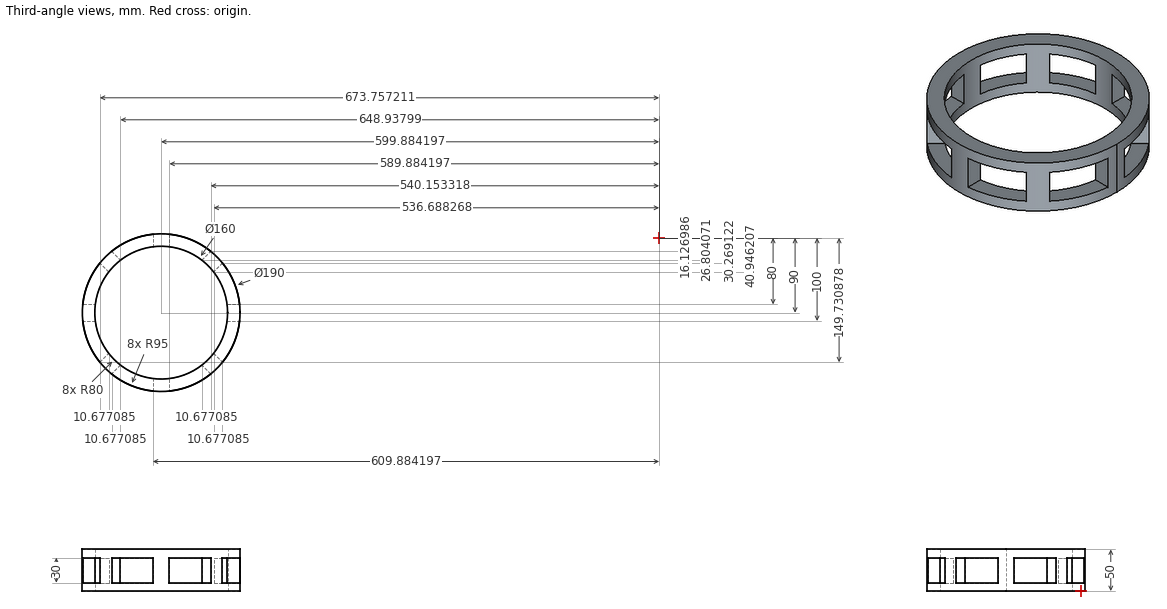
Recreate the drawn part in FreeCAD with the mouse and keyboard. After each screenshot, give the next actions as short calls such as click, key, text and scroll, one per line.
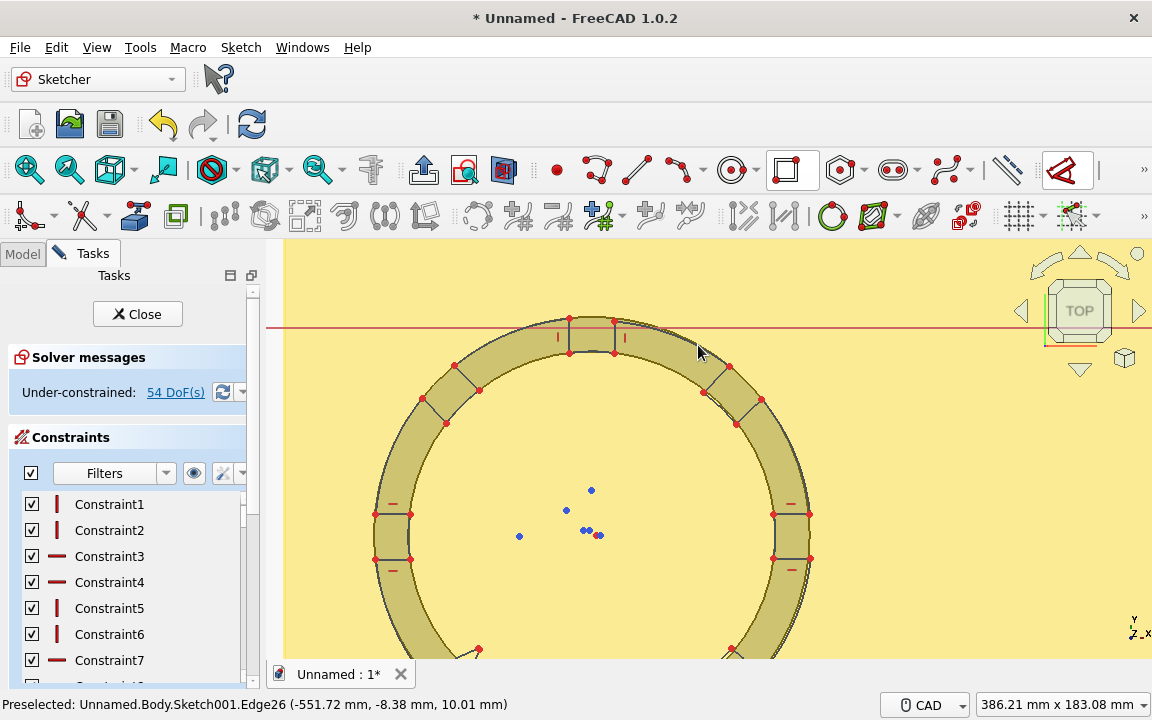
scroll(700, 345, down, 3)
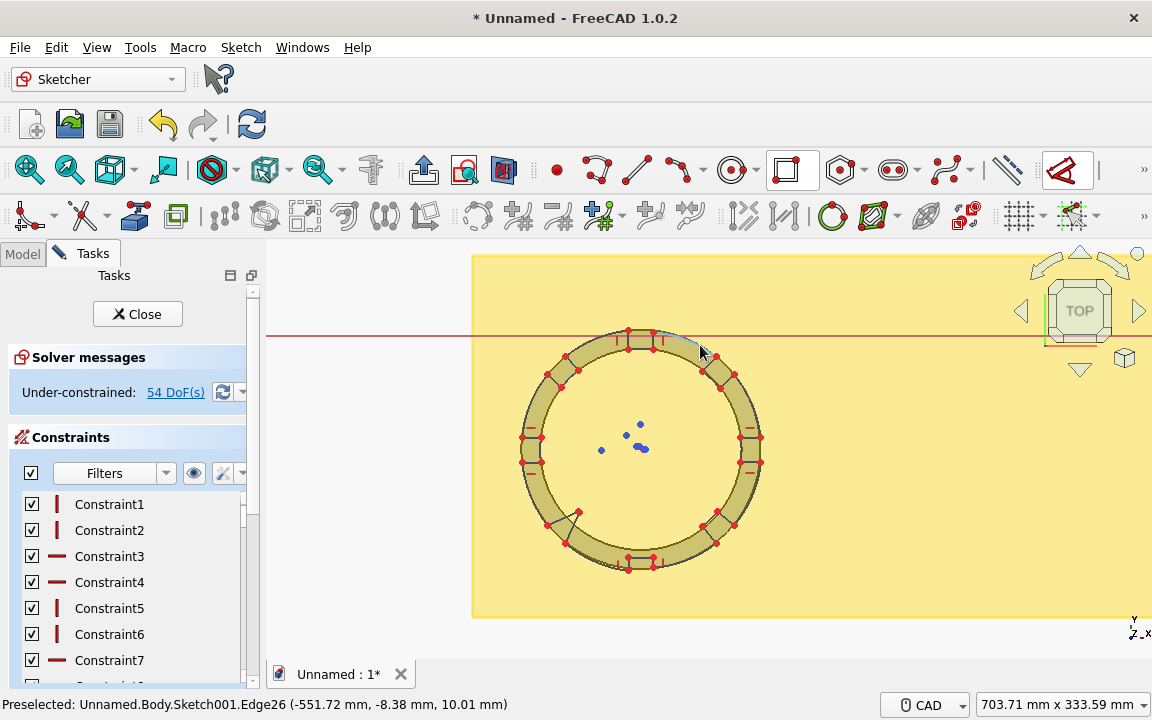
scroll(579, 512, up, 15)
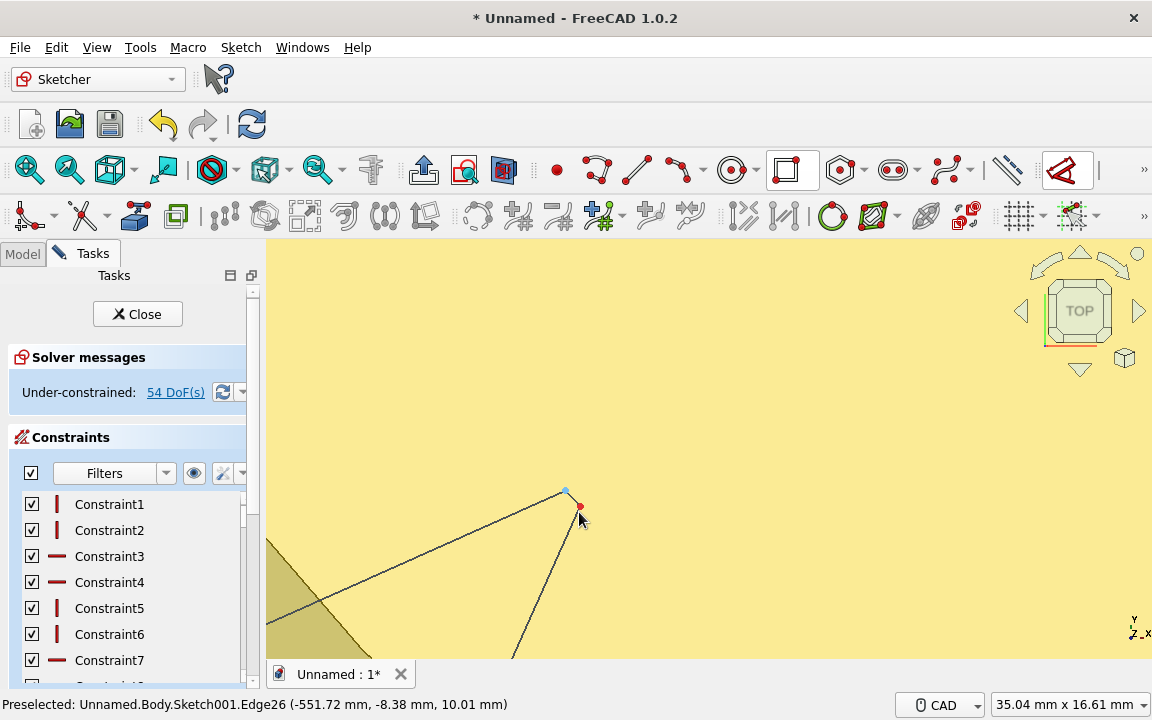
click(573, 499)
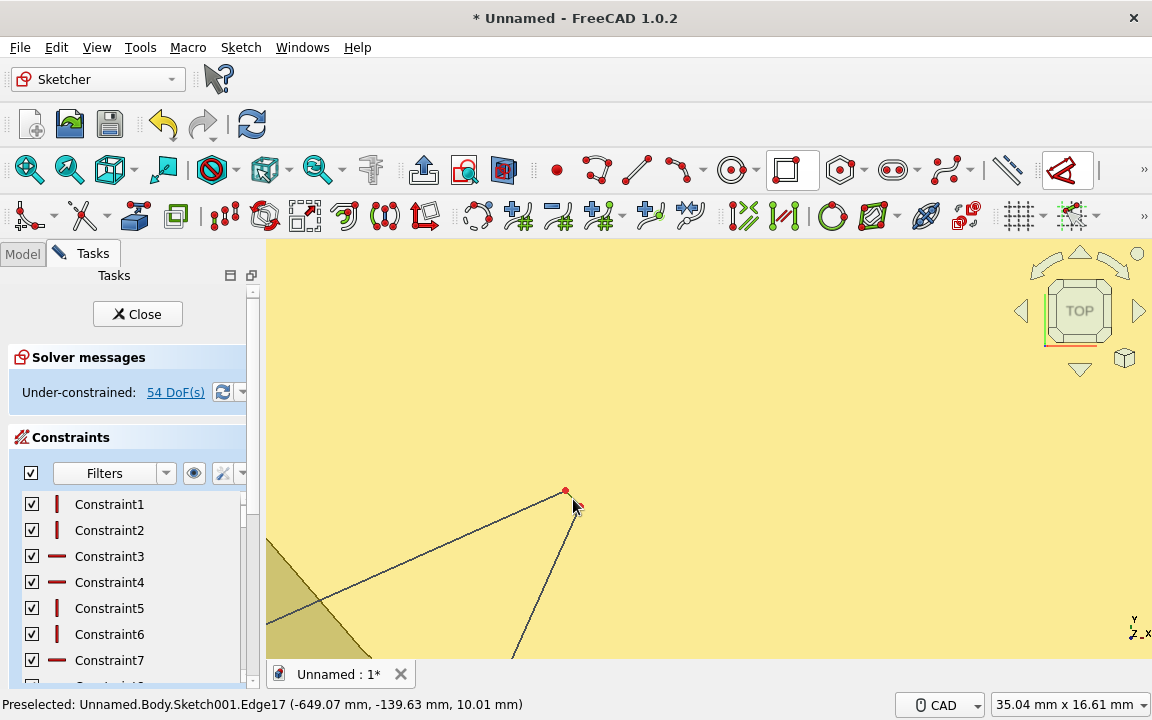
scroll(579, 512, down, 15)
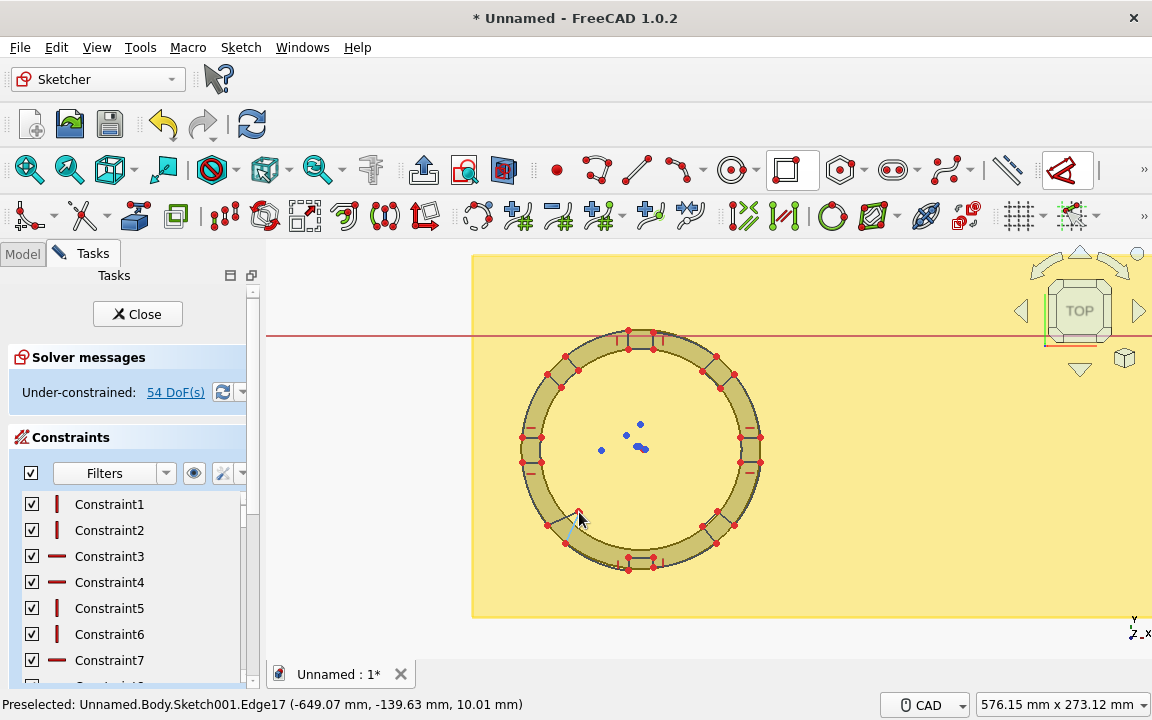
scroll(646, 349, up, 4)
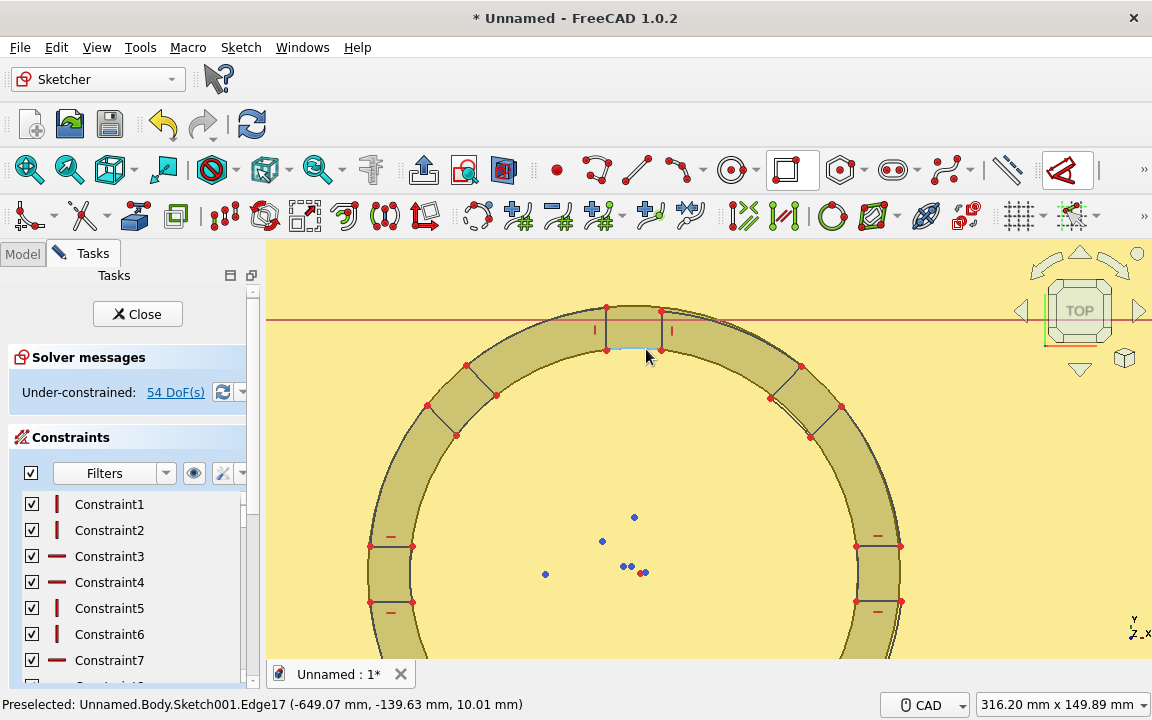
click(645, 348)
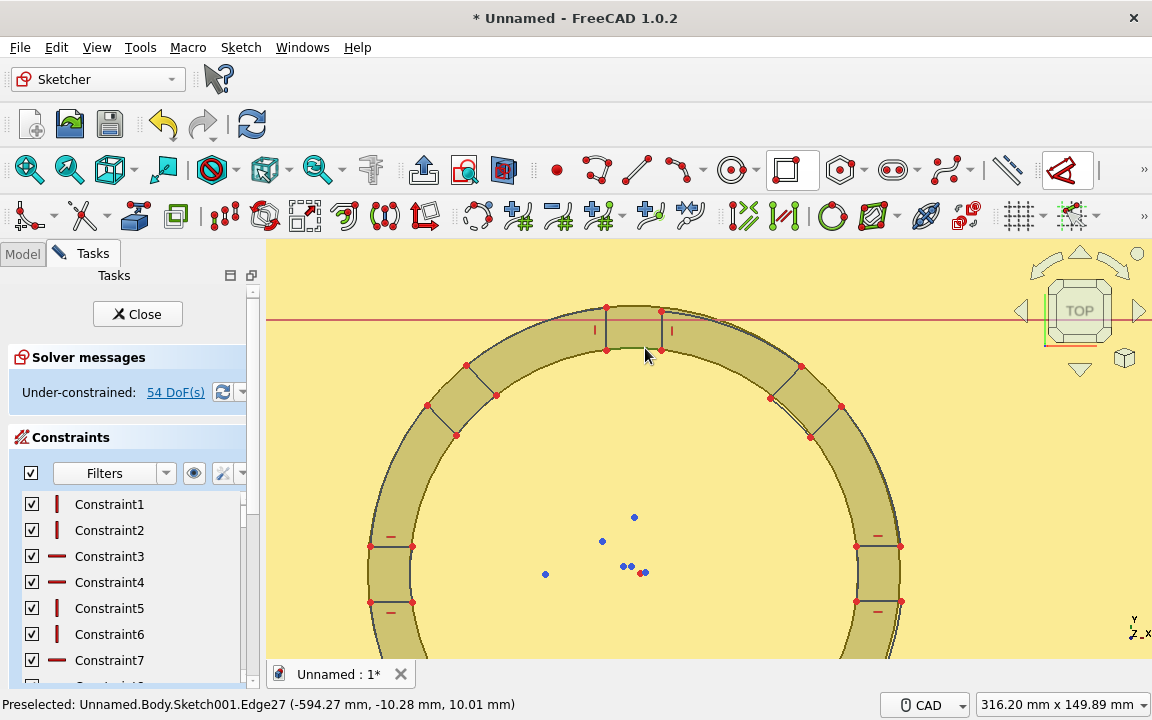
key(c)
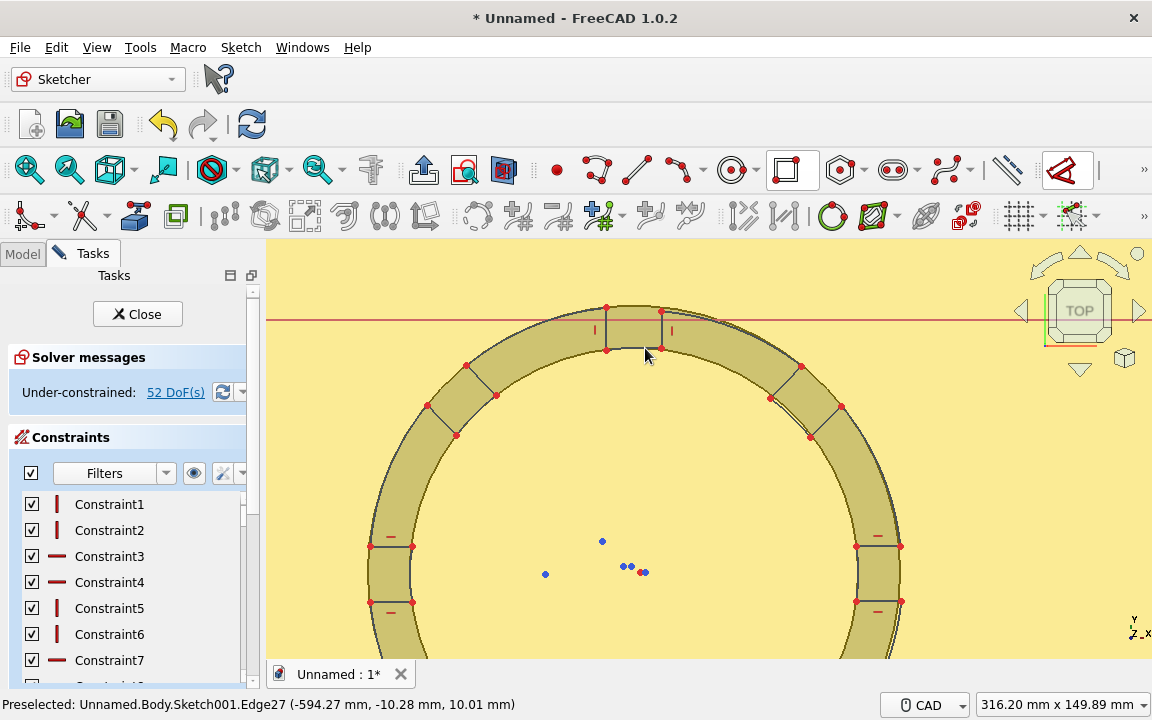
scroll(646, 349, down, 4)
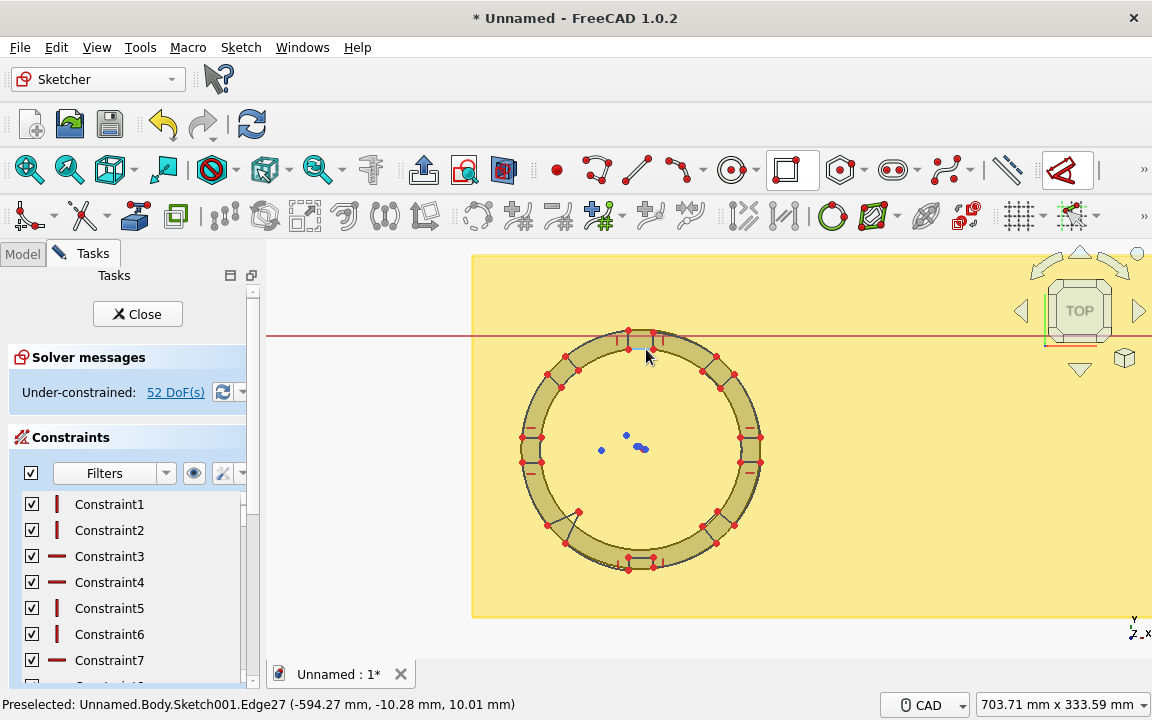
scroll(579, 512, up, 15)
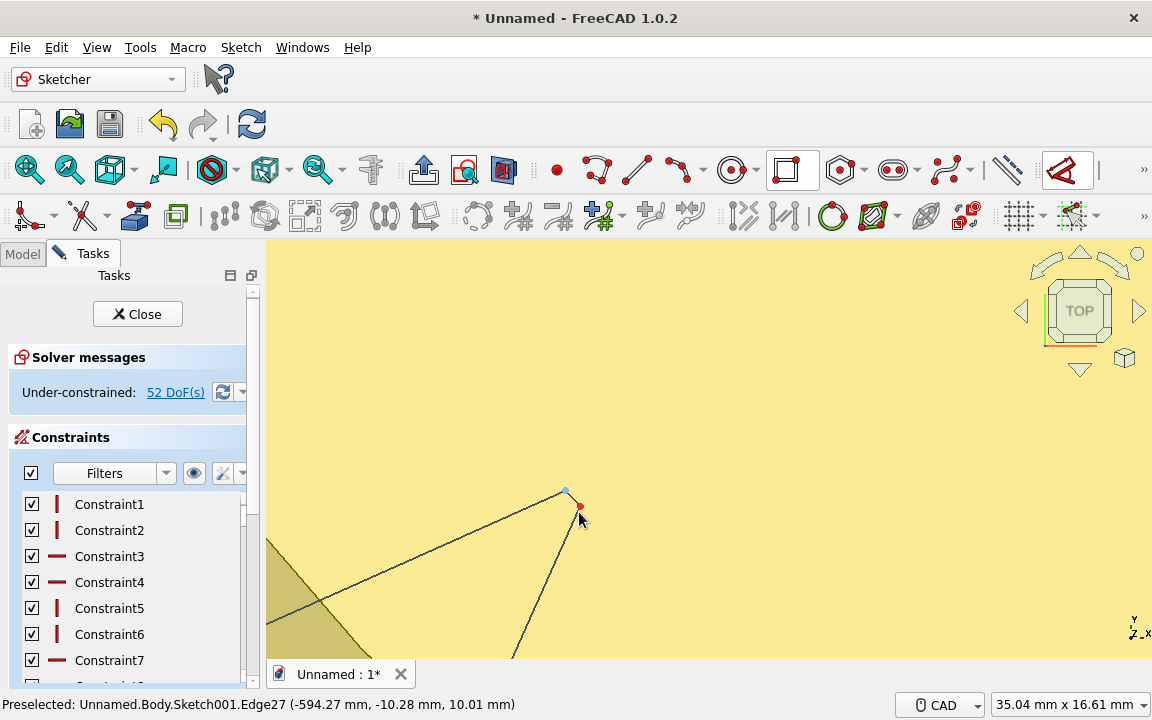
click(573, 499)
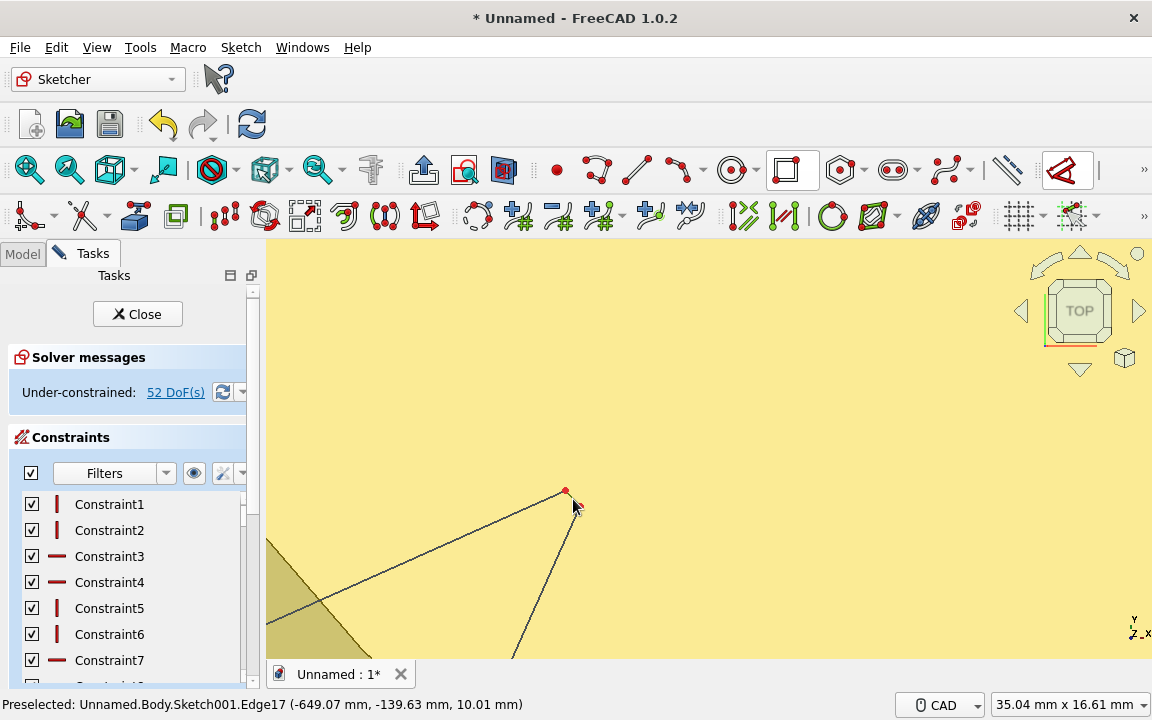
scroll(579, 512, down, 15)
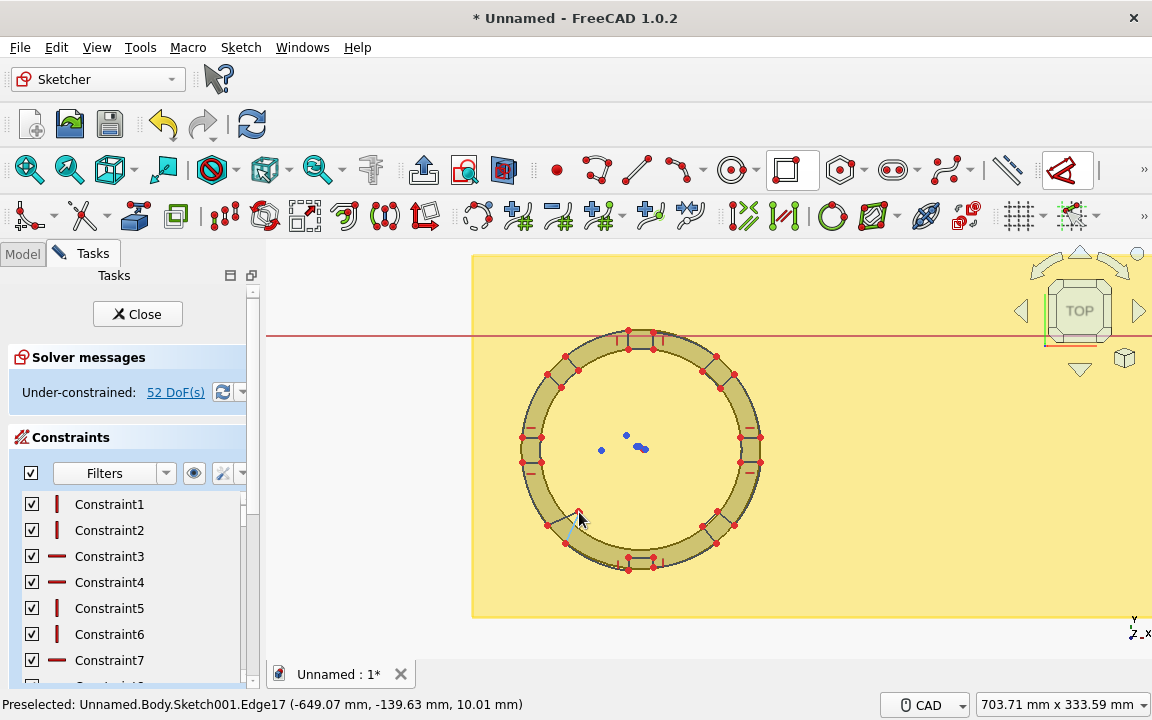
scroll(608, 335, up, 12)